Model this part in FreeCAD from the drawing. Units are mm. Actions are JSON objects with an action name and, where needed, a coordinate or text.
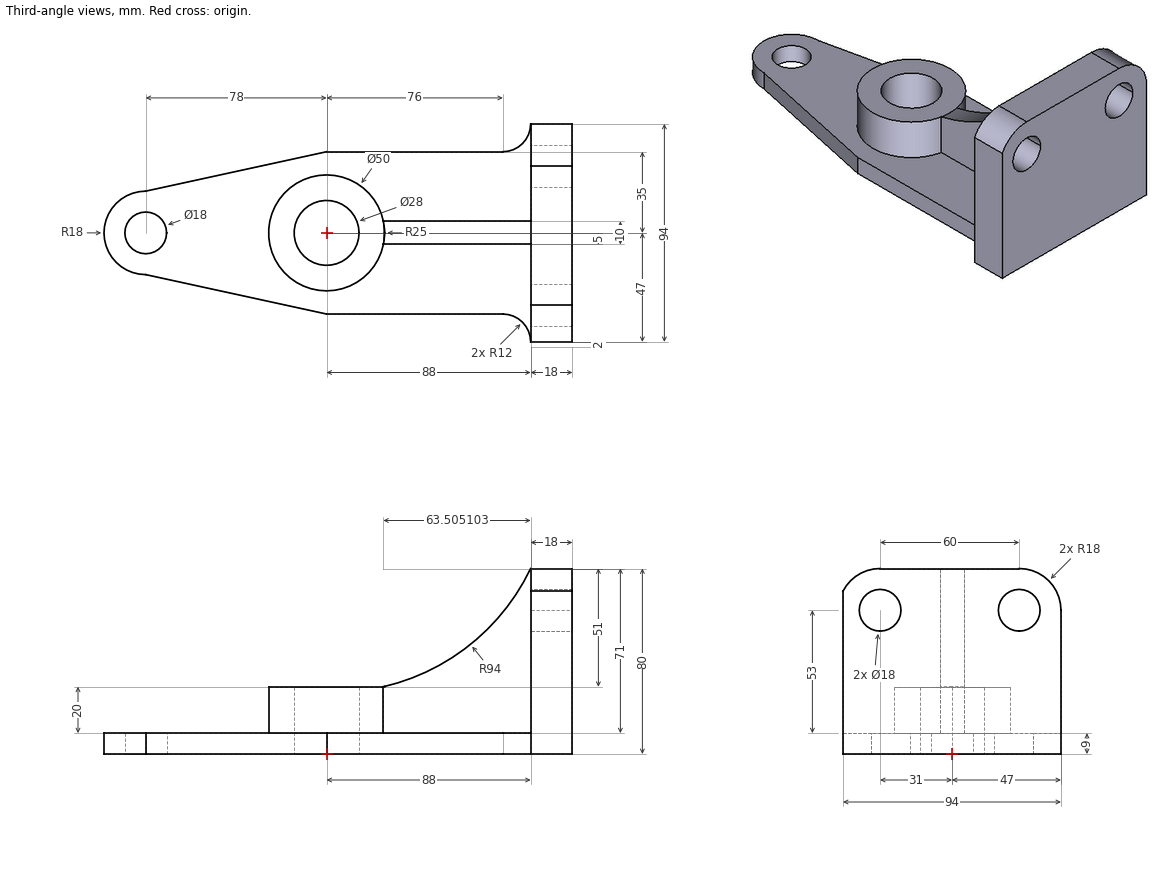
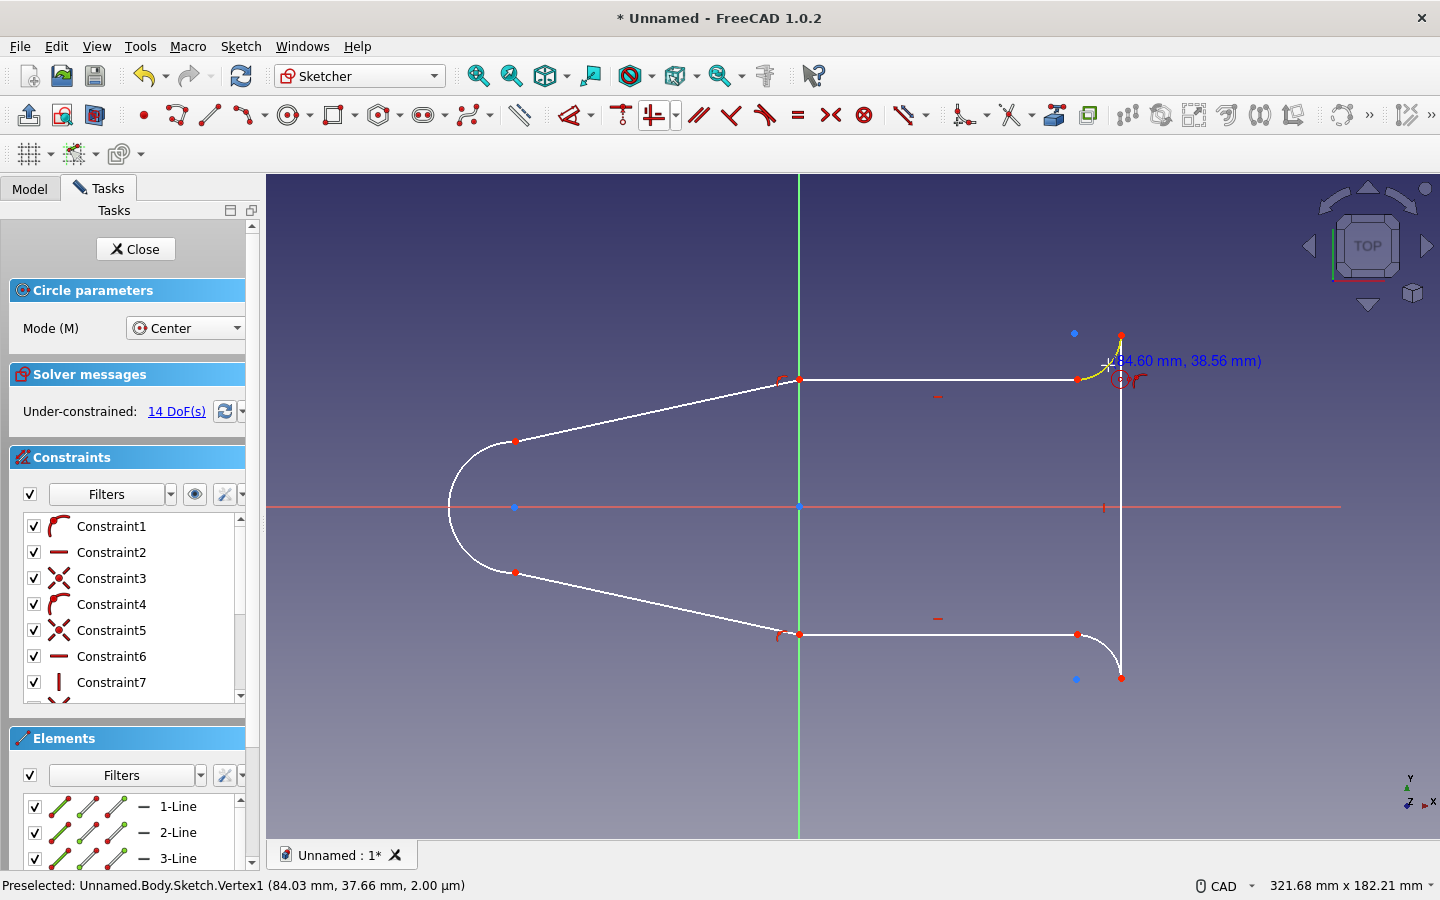
{"action": "left_click", "coordinate": [515, 507]}
{"action": "left_click", "coordinate": [538, 483]}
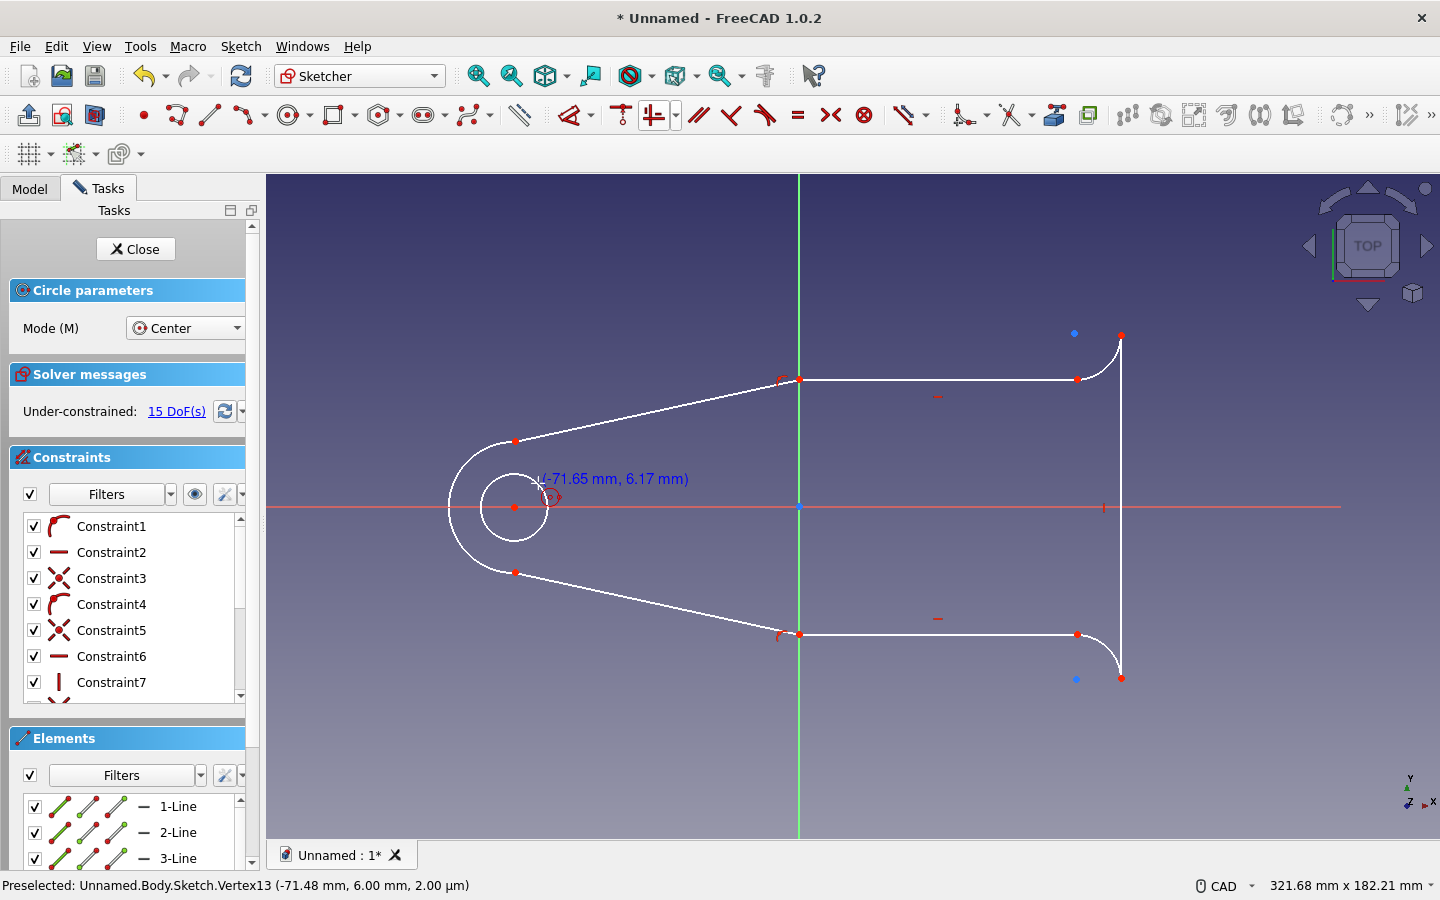
{"action": "left_click", "coordinate": [799, 507]}
{"action": "left_click", "coordinate": [836, 470]}
{"action": "key", "text": "Escape"}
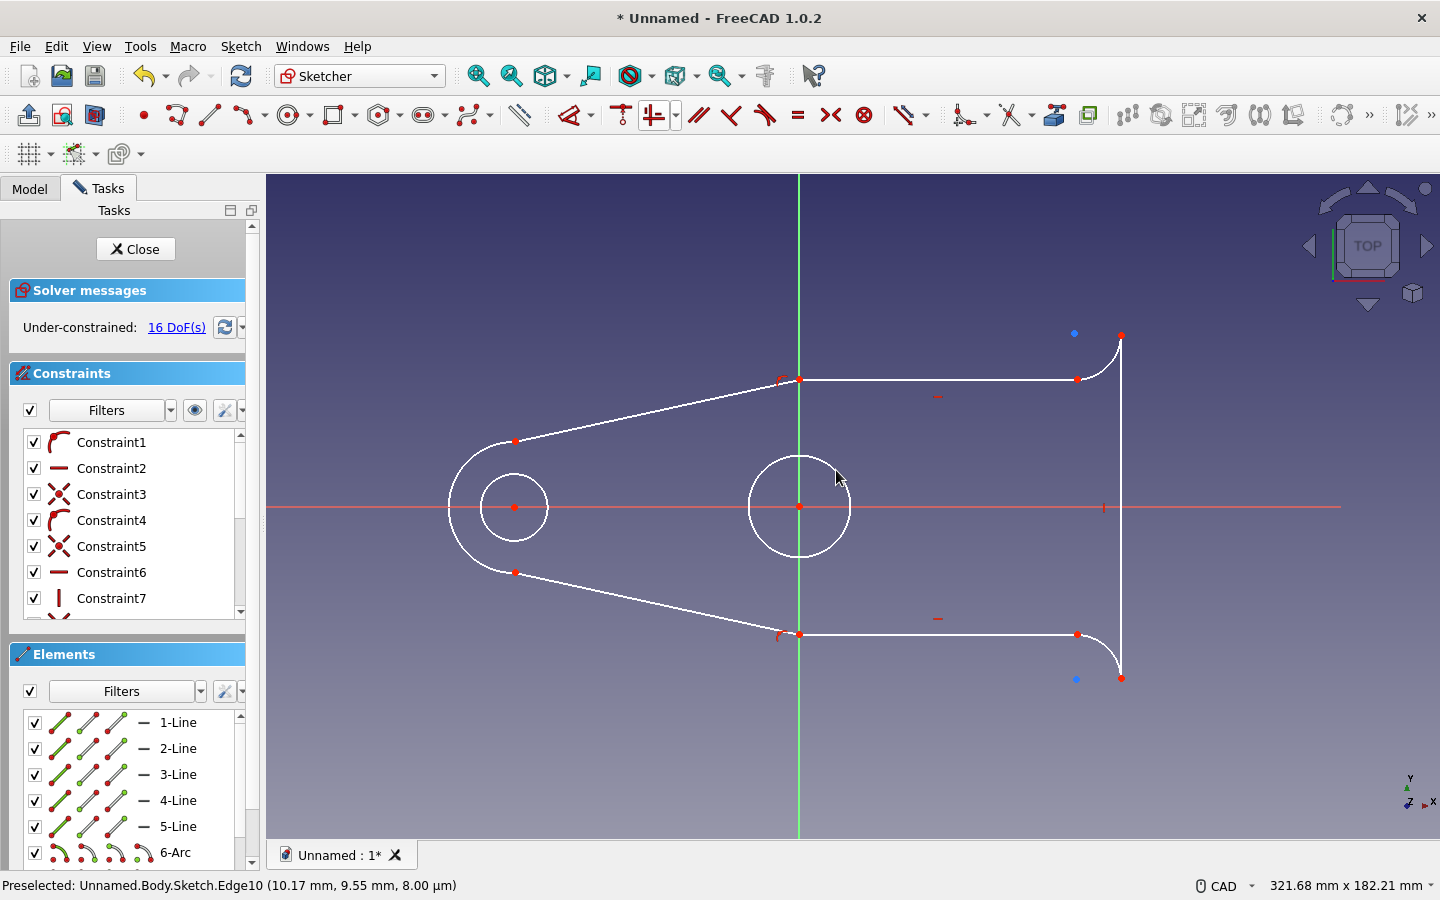
{"action": "left_click", "coordinate": [994, 380]}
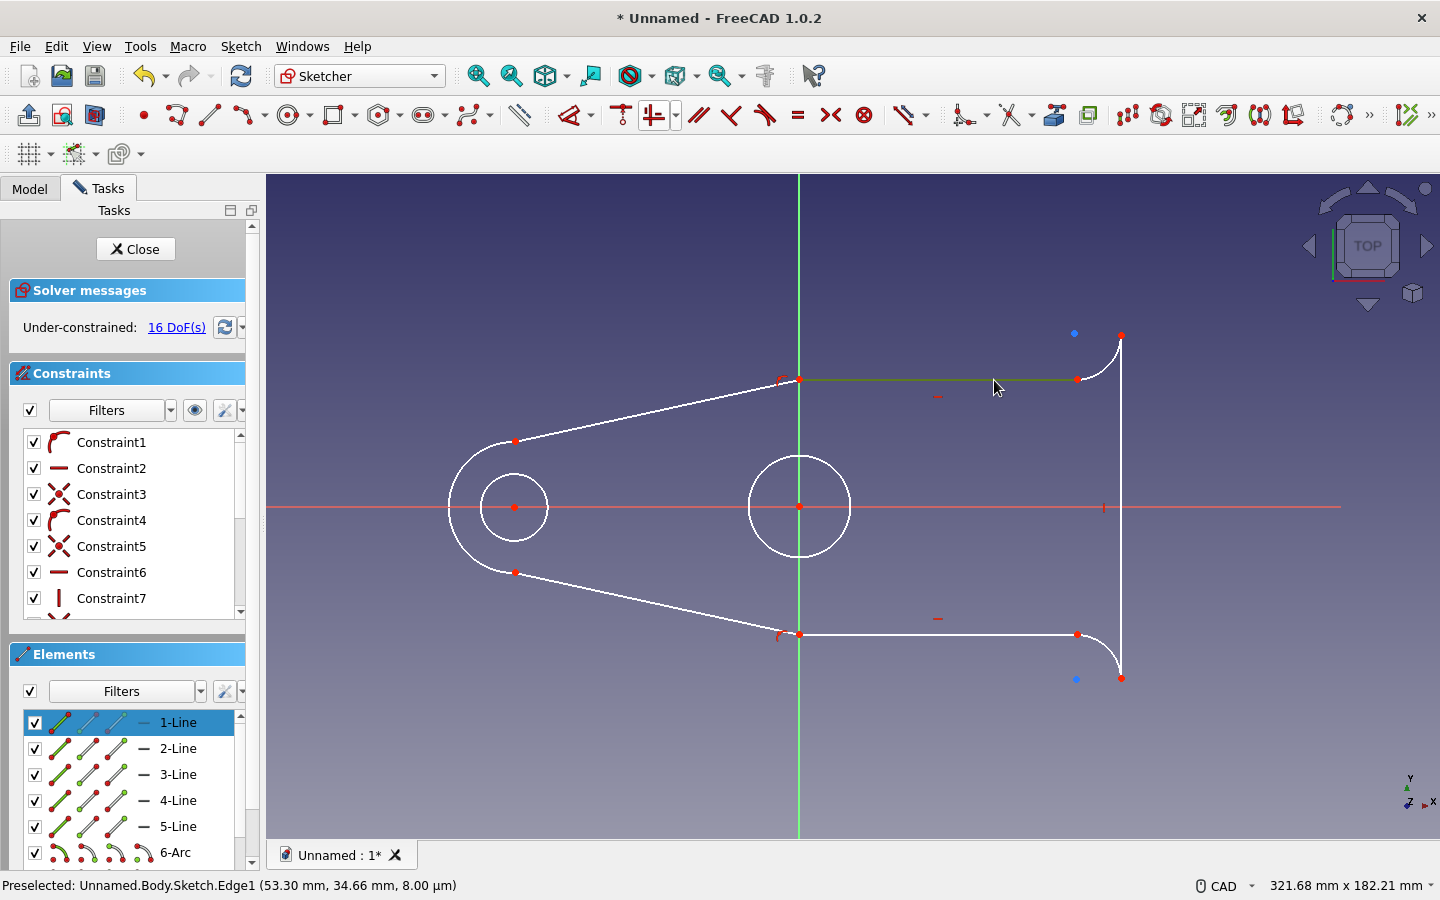
{"action": "left_click", "coordinate": [1097, 375]}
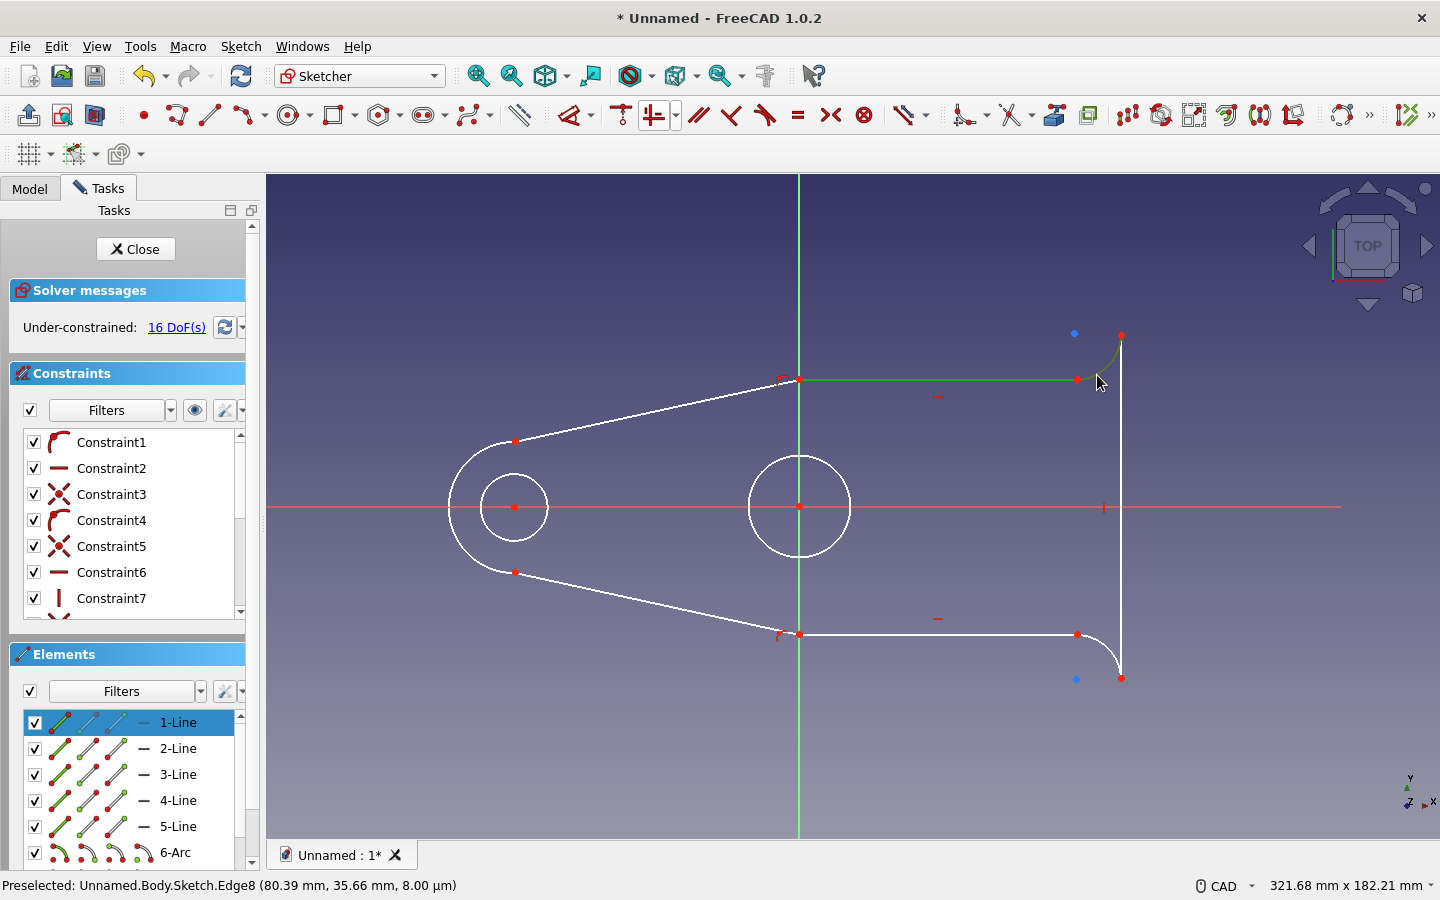
{"action": "left_click", "coordinate": [765, 116]}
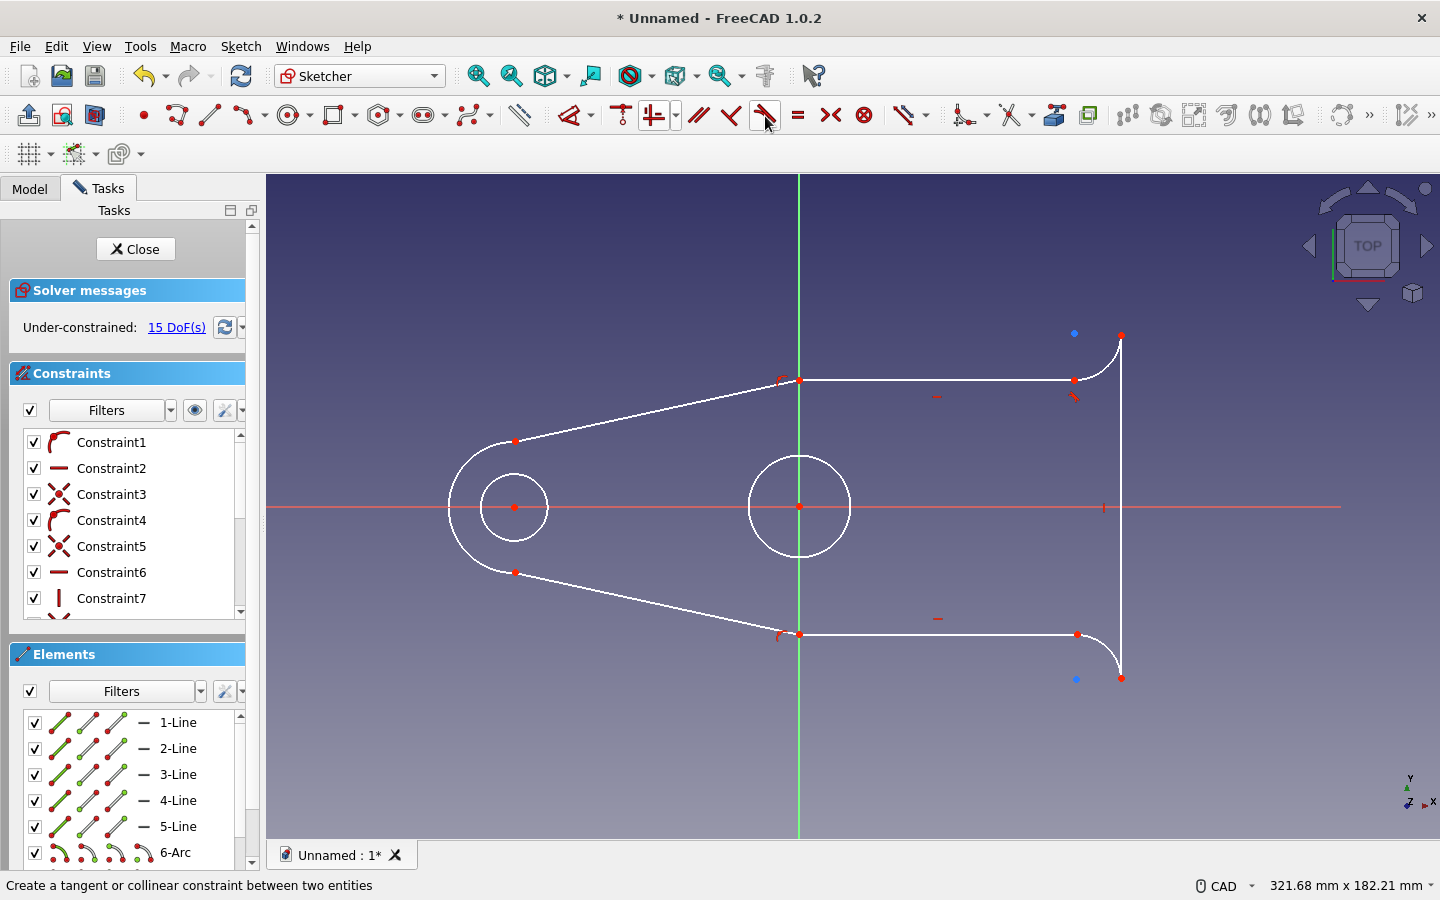
{"action": "left_click", "coordinate": [883, 635]}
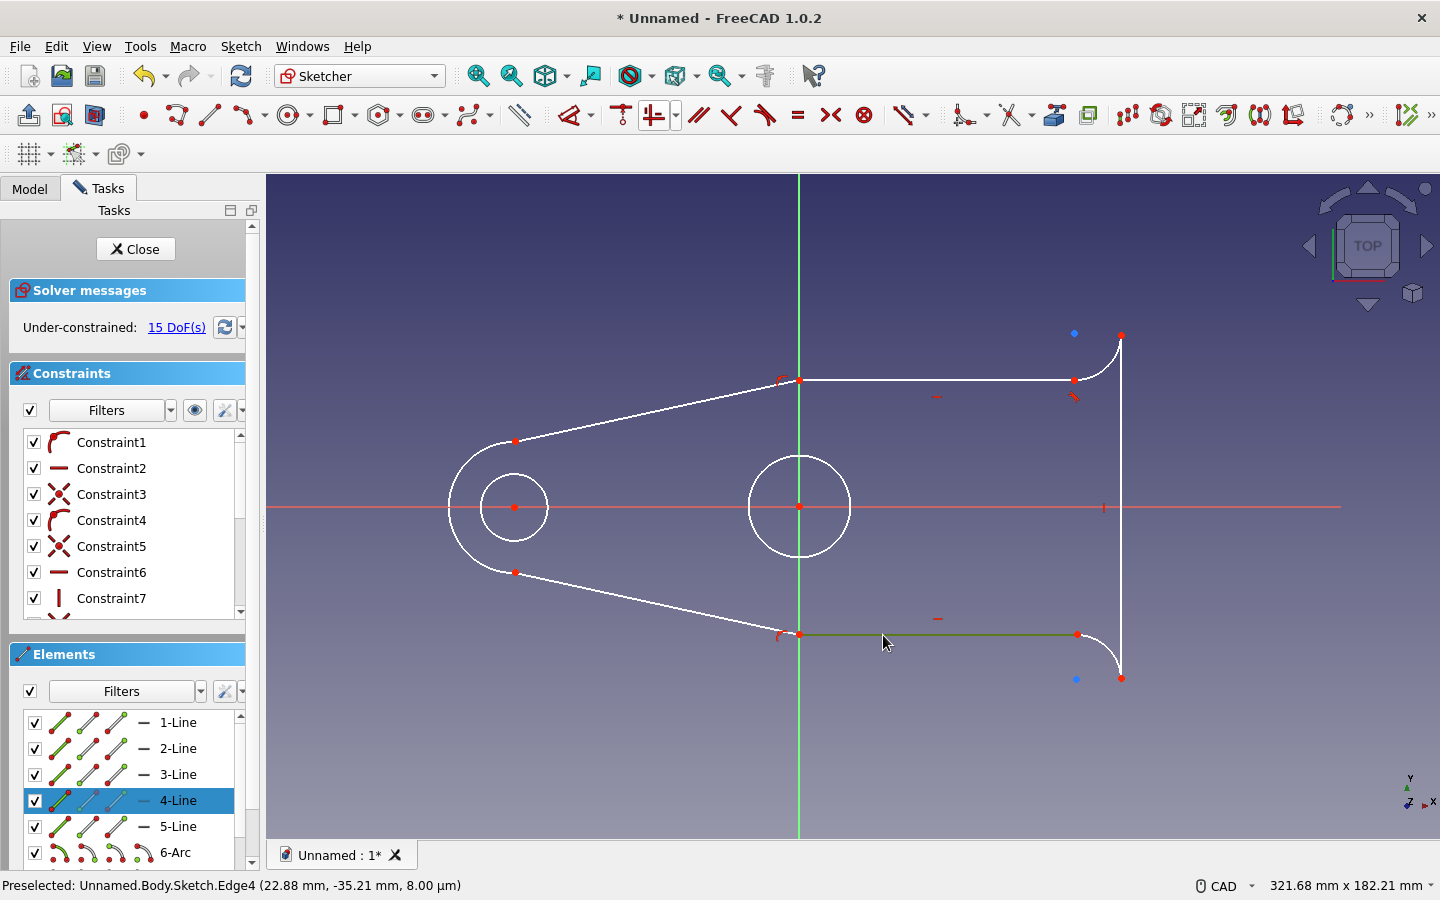
{"action": "left_click", "coordinate": [1097, 640]}